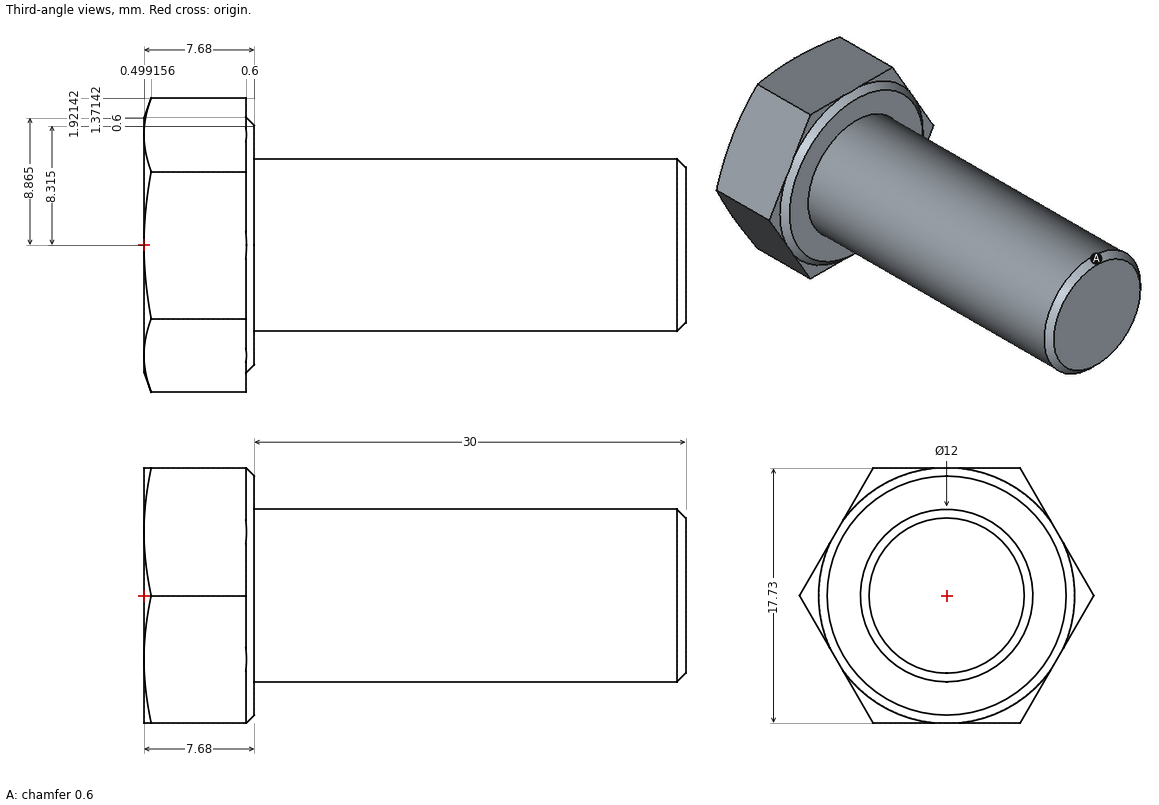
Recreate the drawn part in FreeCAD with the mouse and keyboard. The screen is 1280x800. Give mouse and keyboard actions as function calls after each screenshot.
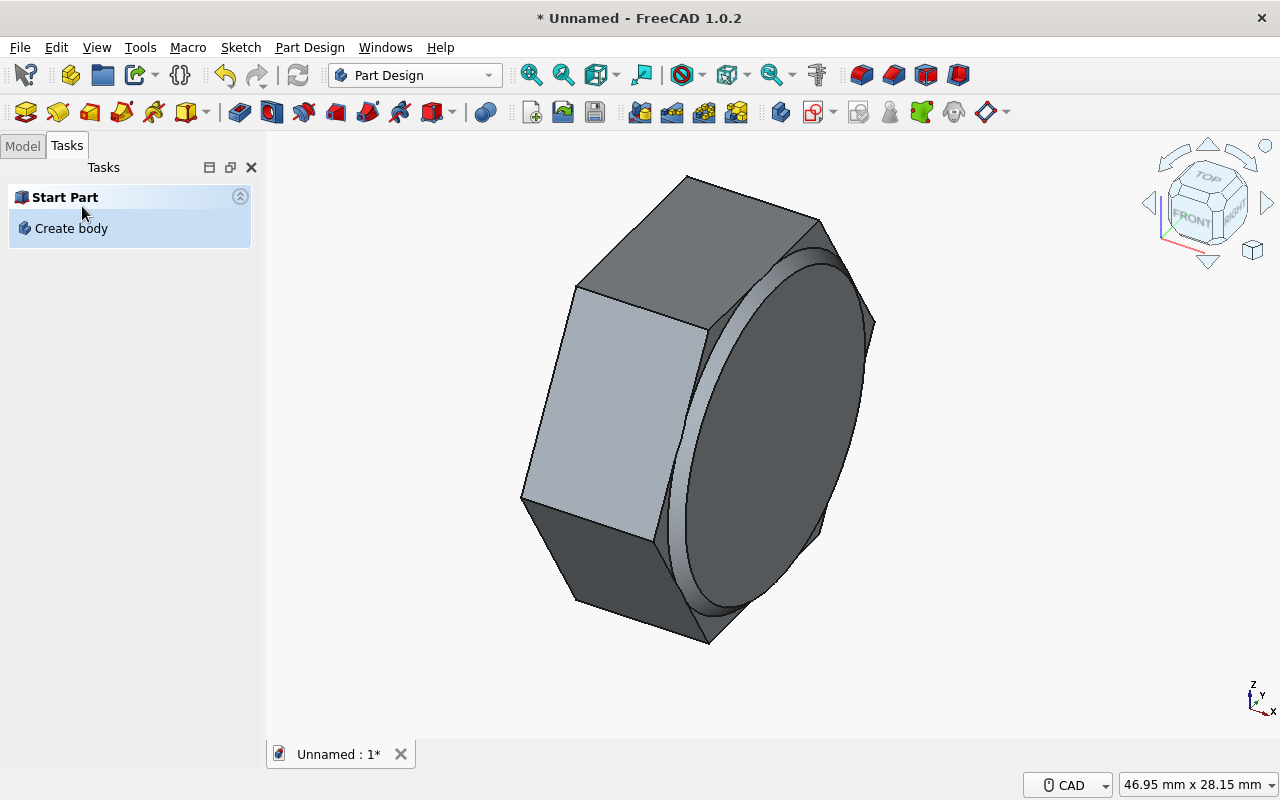
click(532, 76)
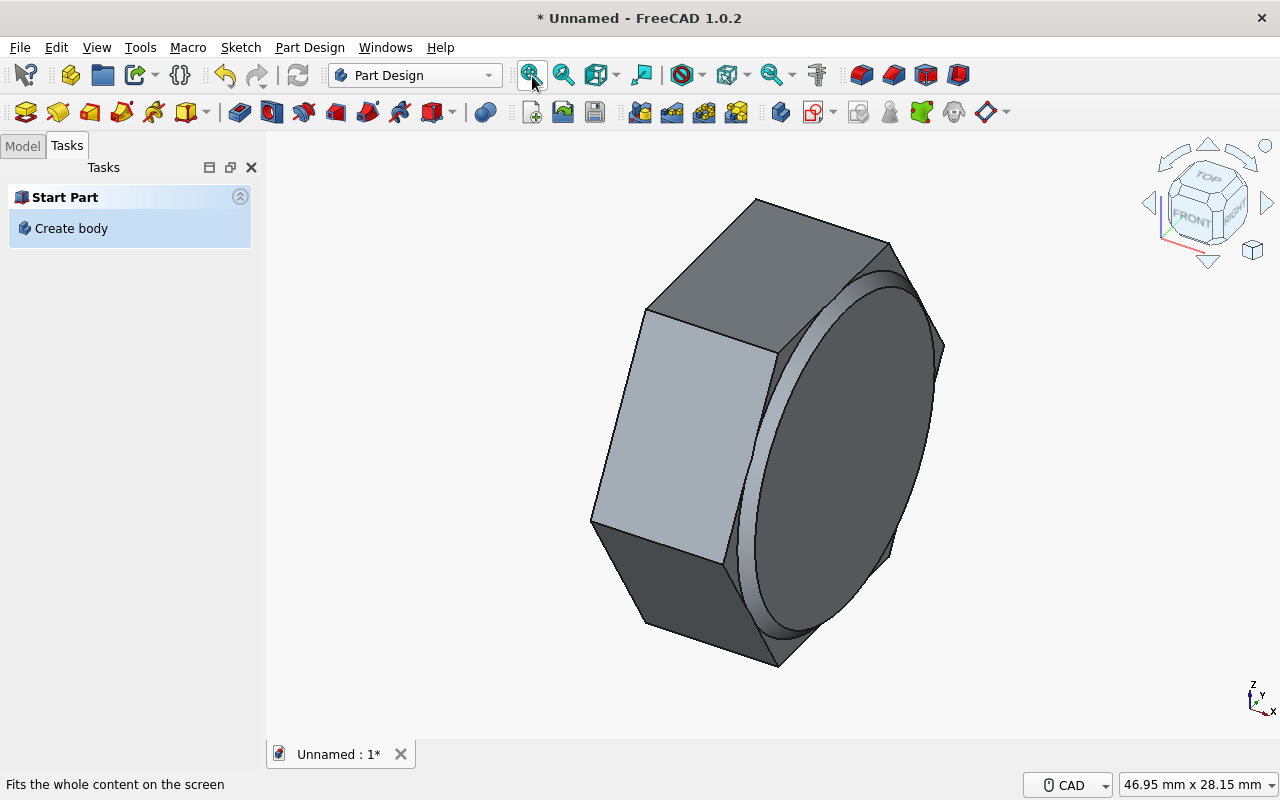
click(814, 112)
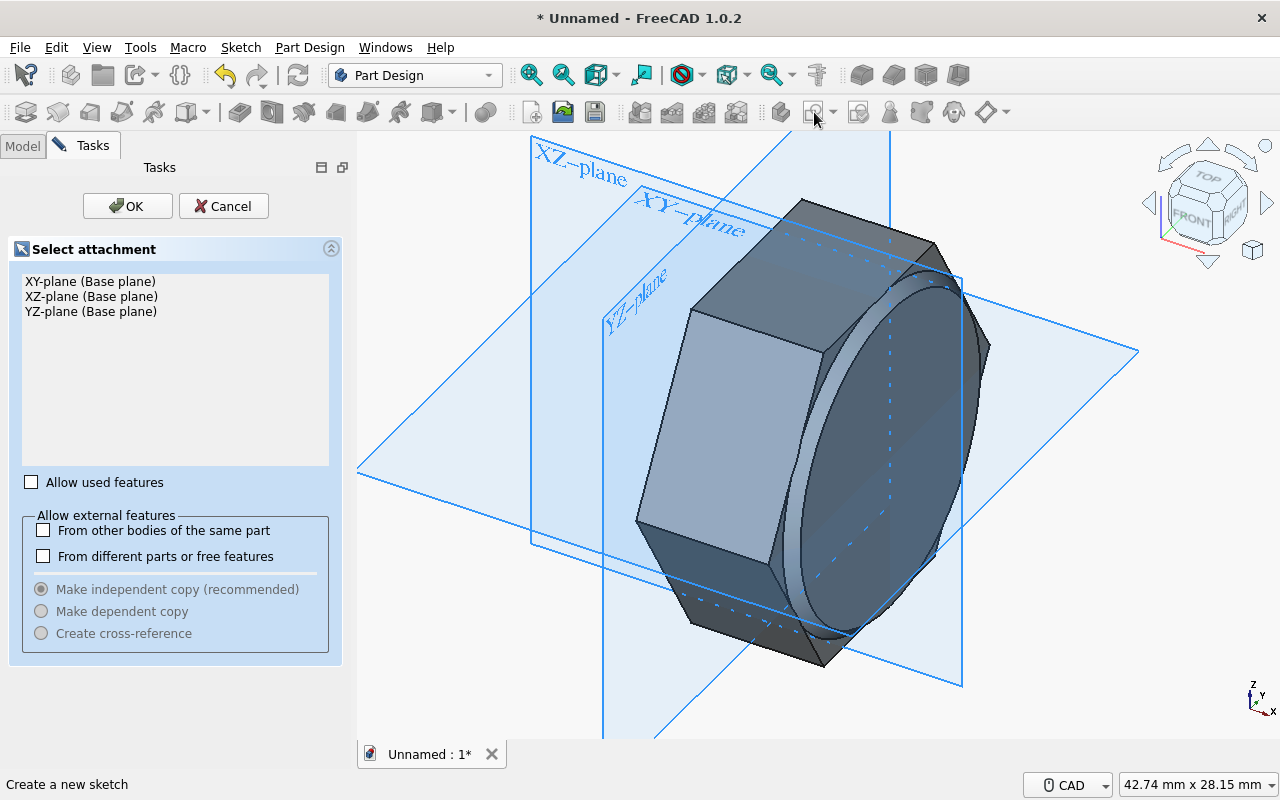
click(82, 282)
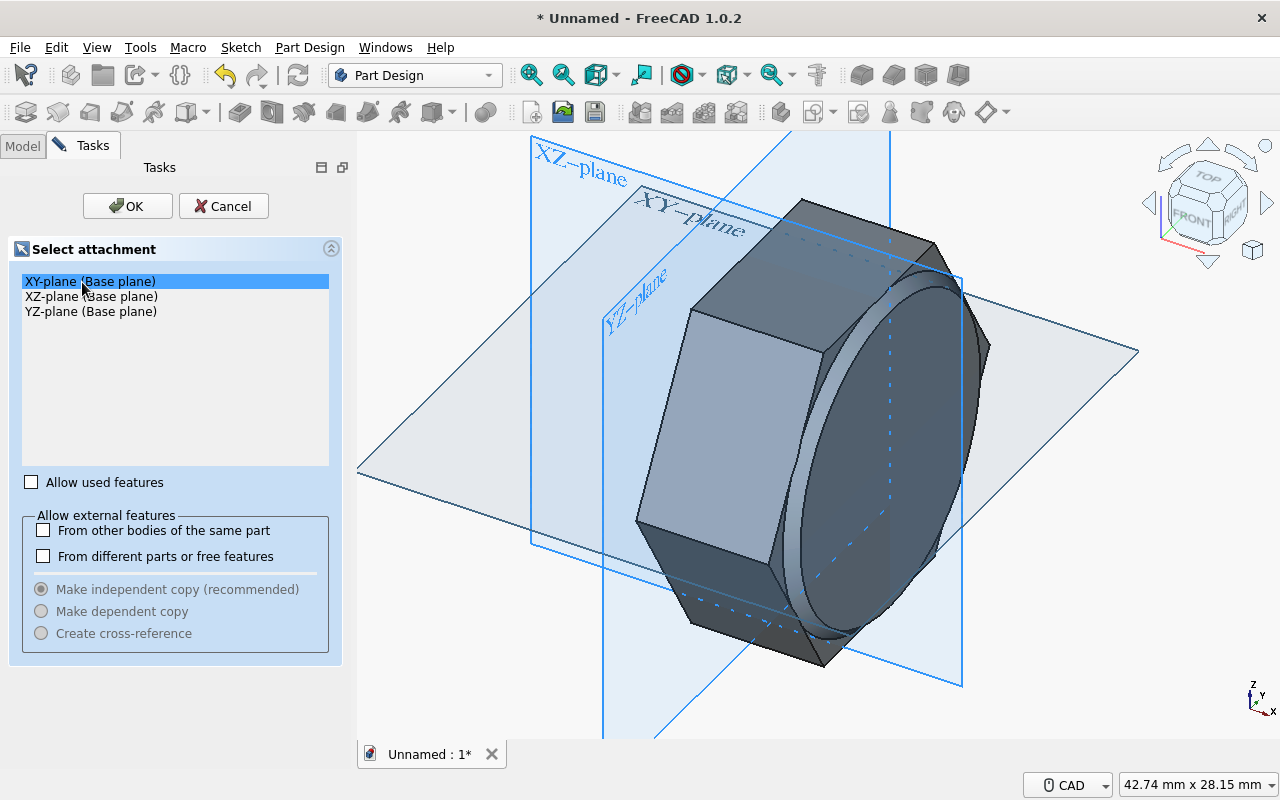
click(128, 206)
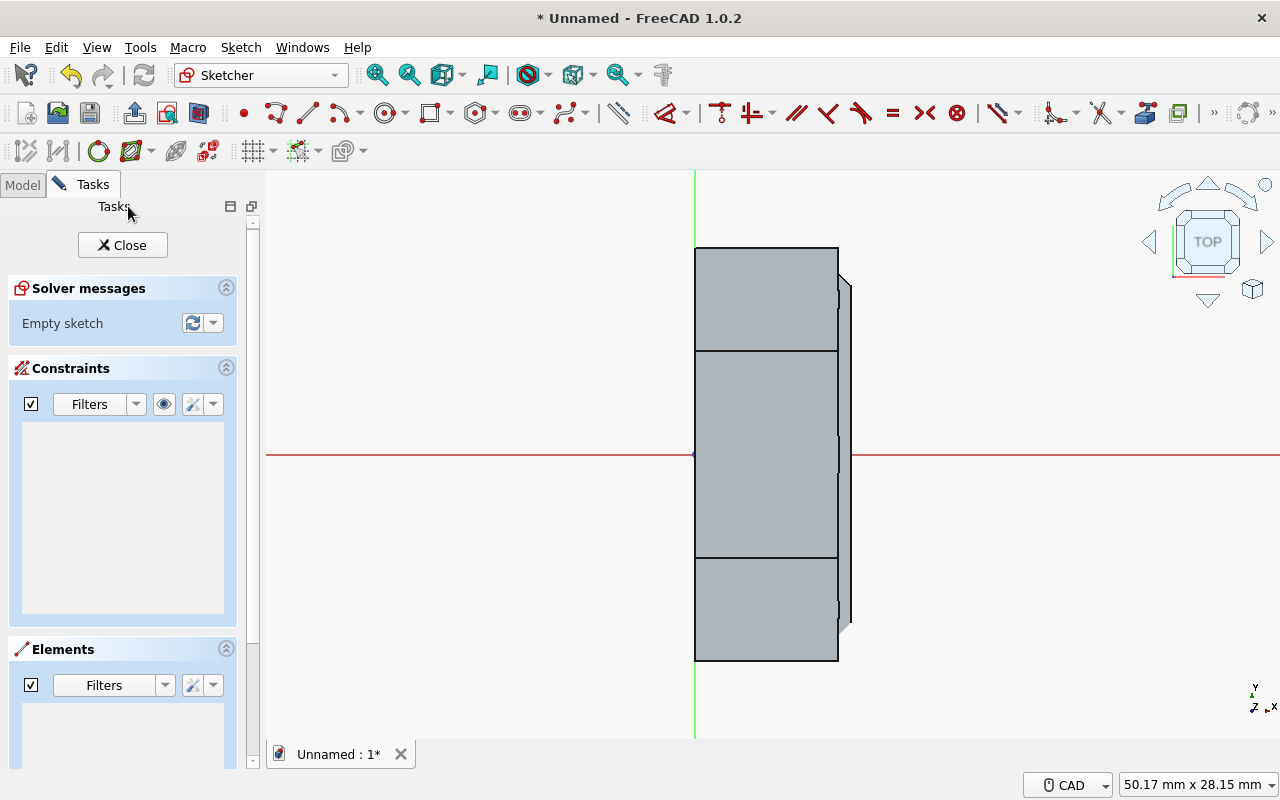
click(200, 114)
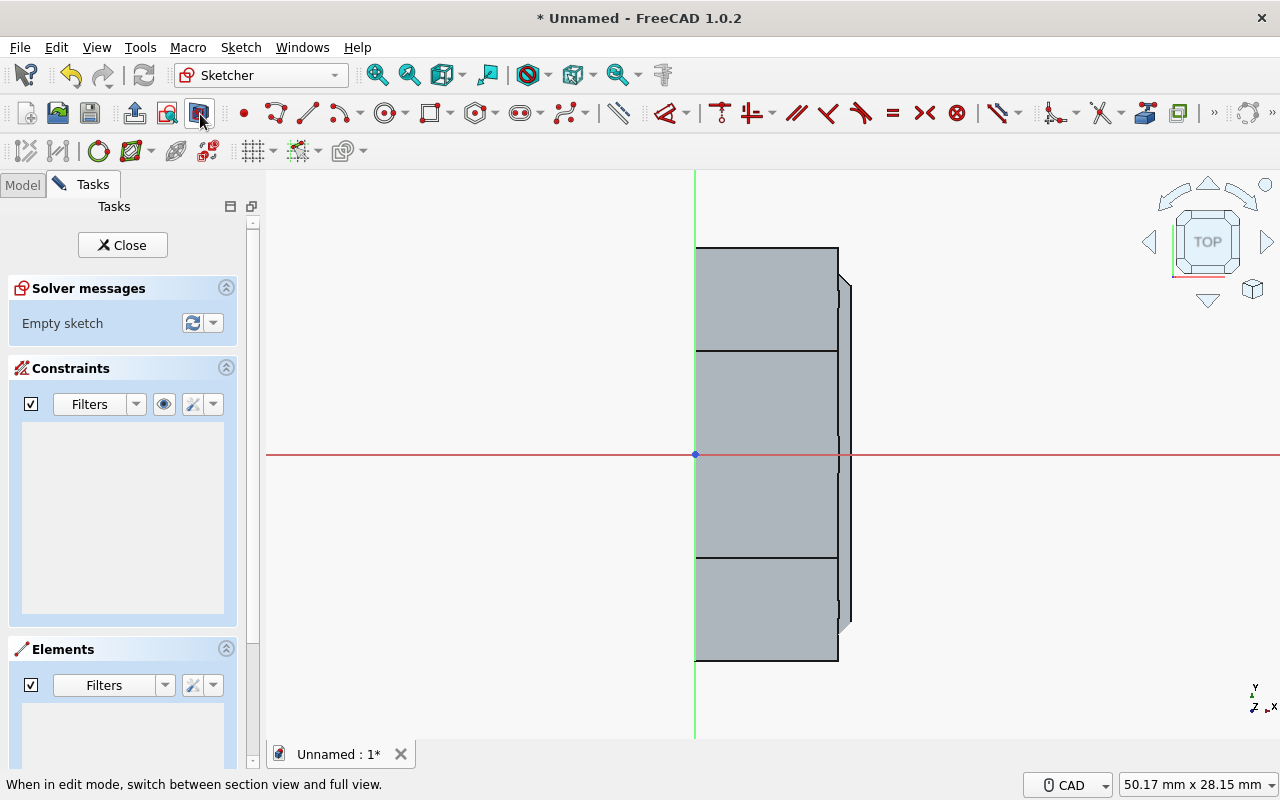
scroll(700, 246, up, 13)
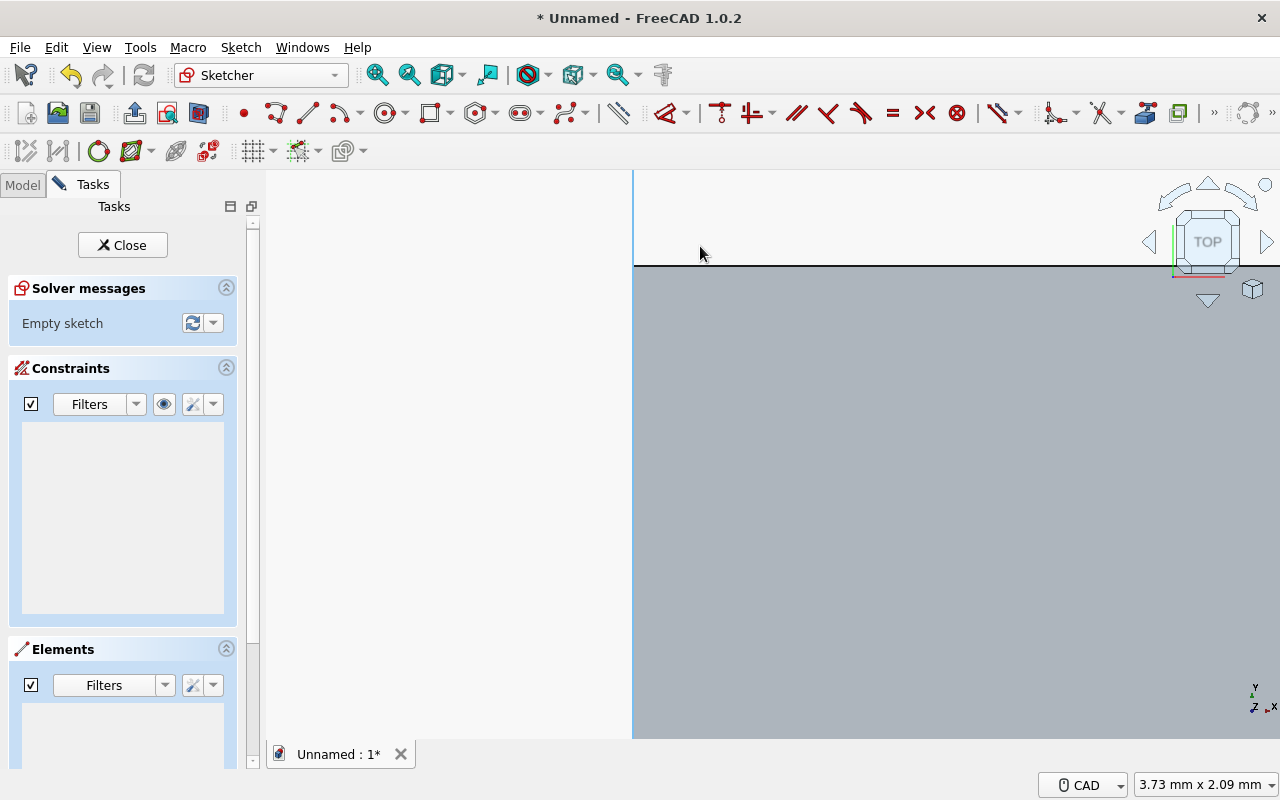
click(276, 114)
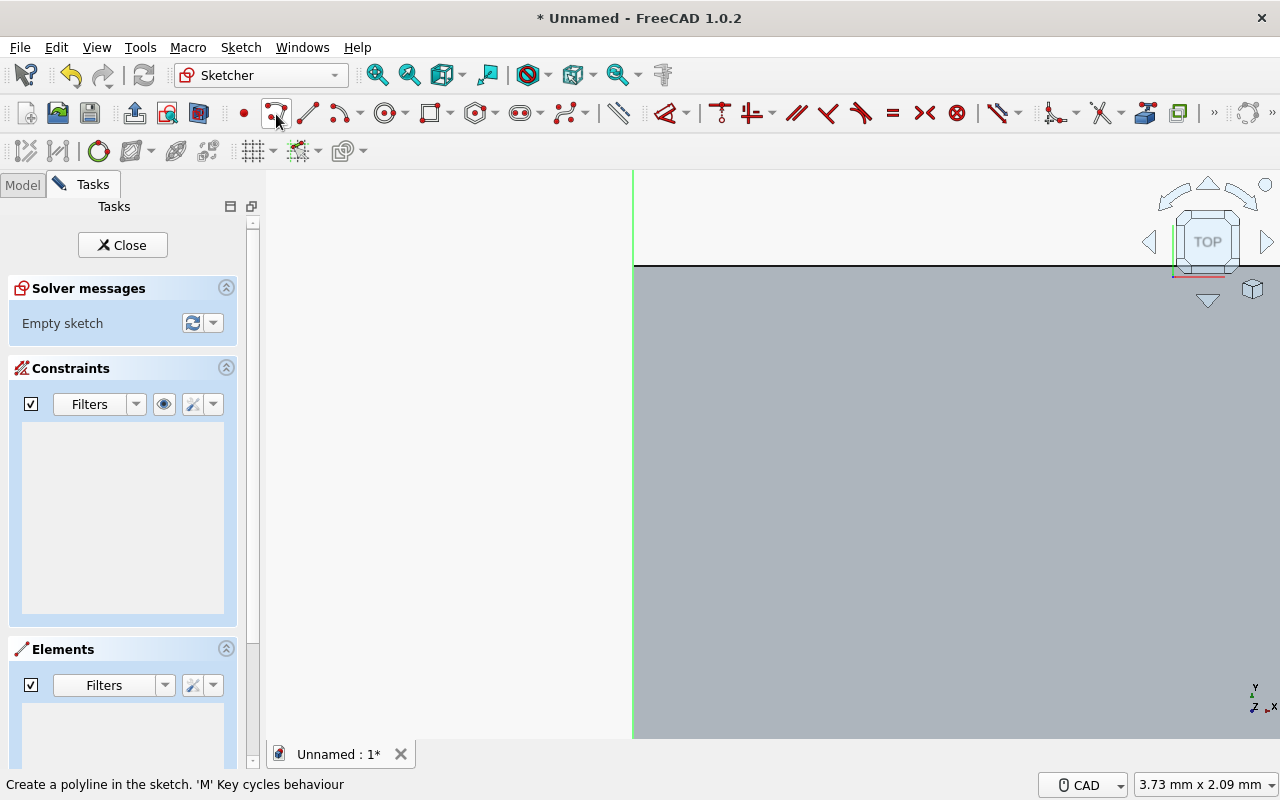
click(633, 639)
click(768, 266)
click(642, 266)
click(633, 640)
key(Escape)
key(Escape)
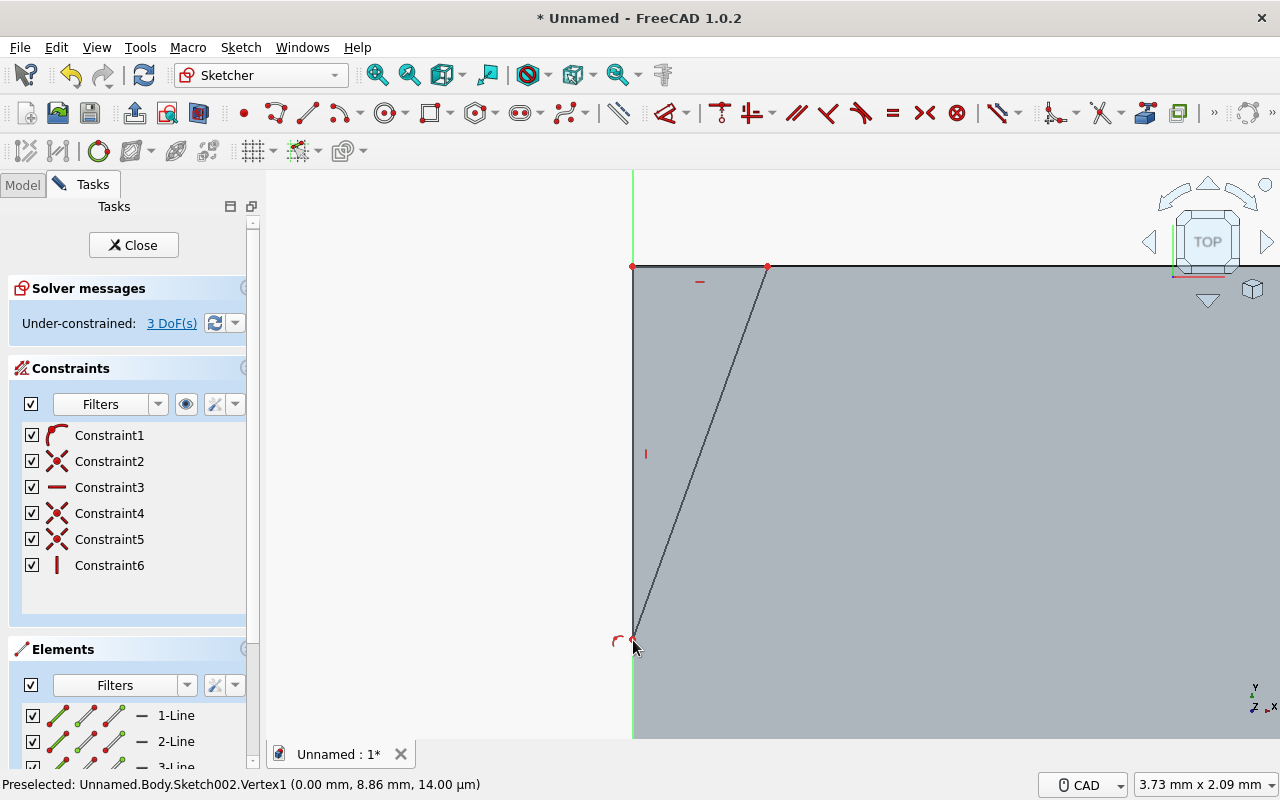
click(666, 114)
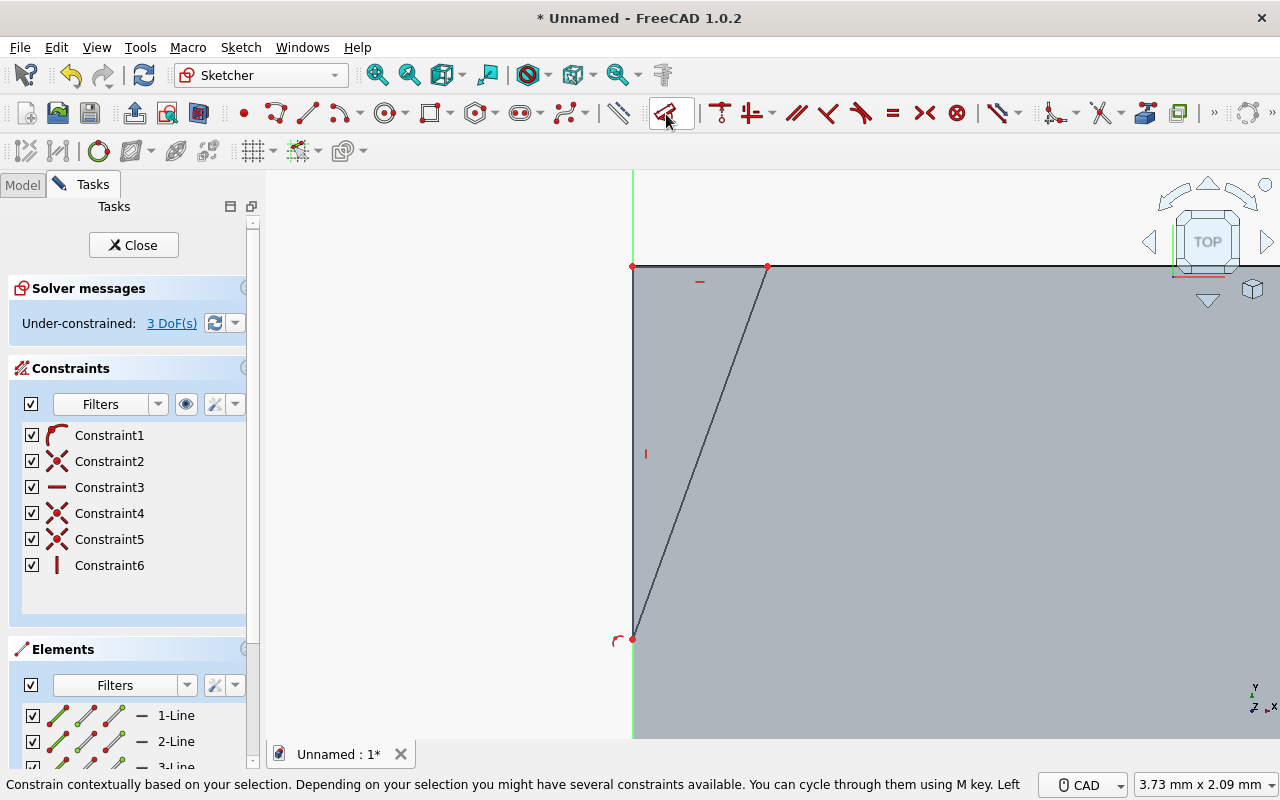
click(633, 640)
click(599, 676)